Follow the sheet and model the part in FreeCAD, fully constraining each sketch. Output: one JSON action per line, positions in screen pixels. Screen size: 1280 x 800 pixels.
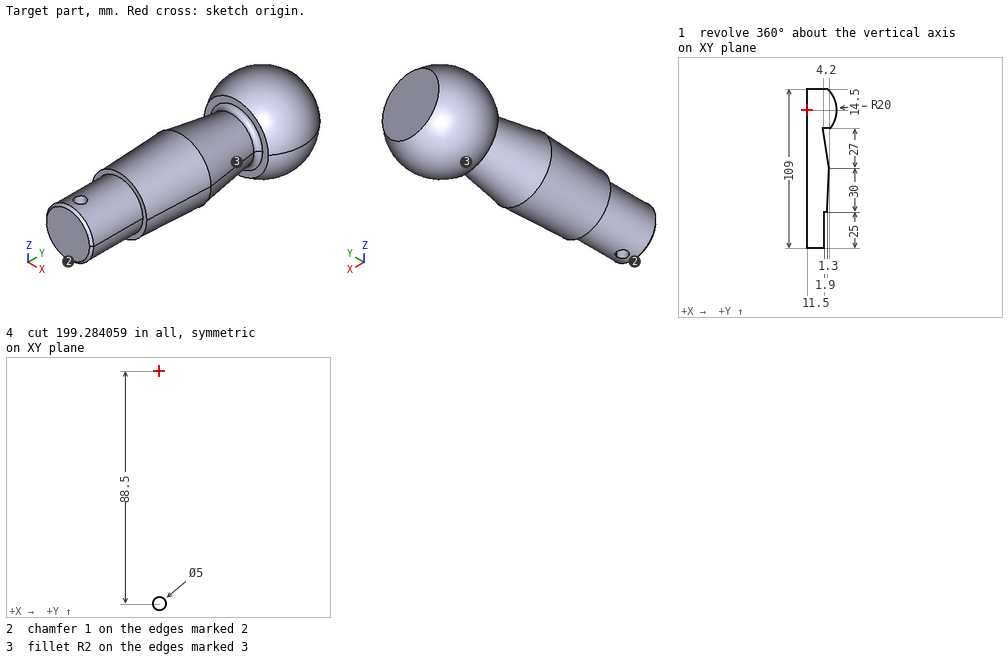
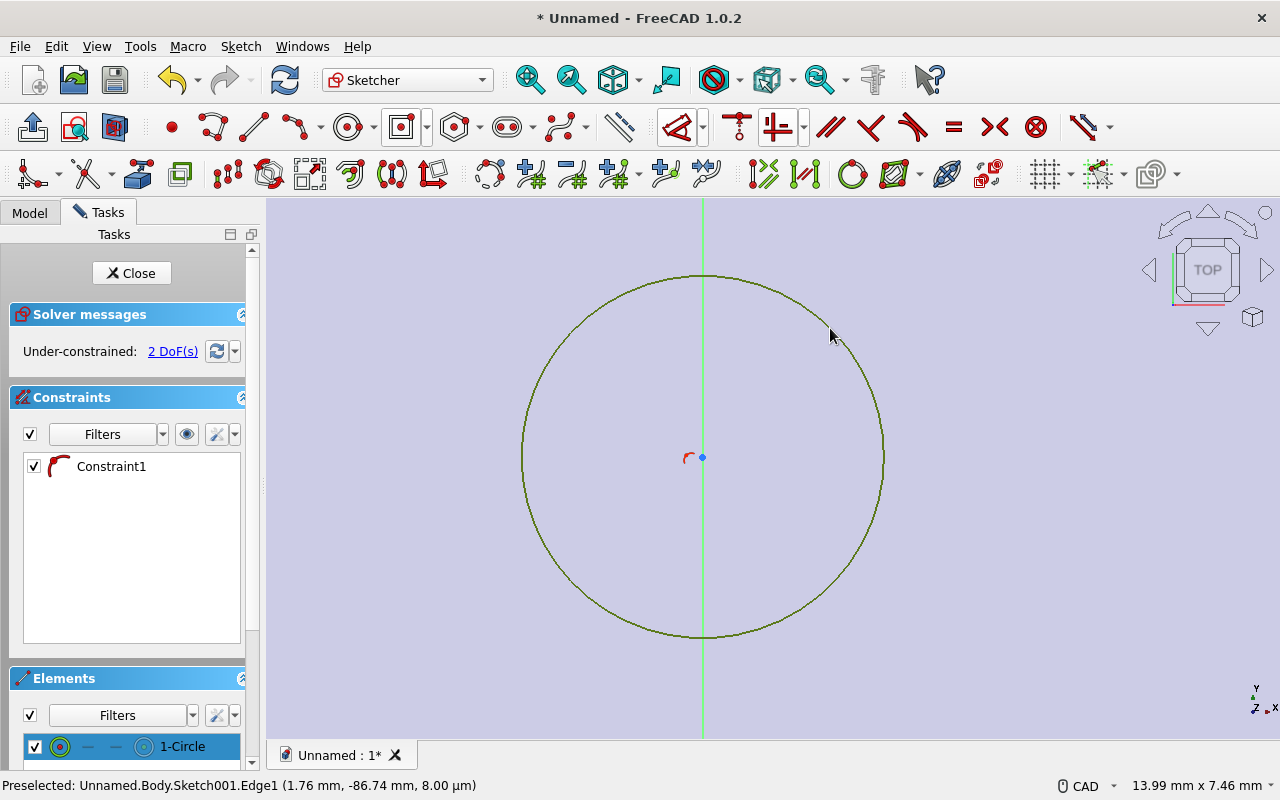
{"action": "left_click", "coordinate": [702, 128]}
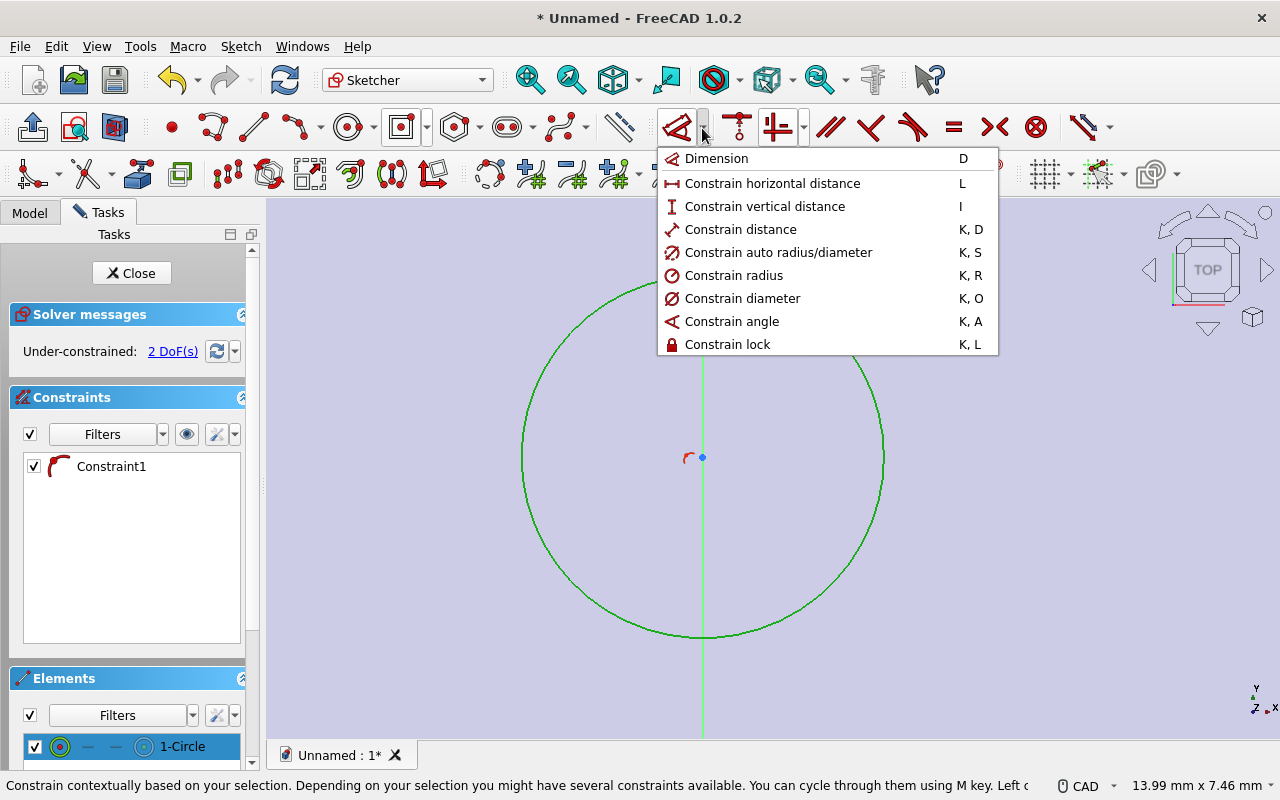
{"action": "left_click", "coordinate": [828, 298]}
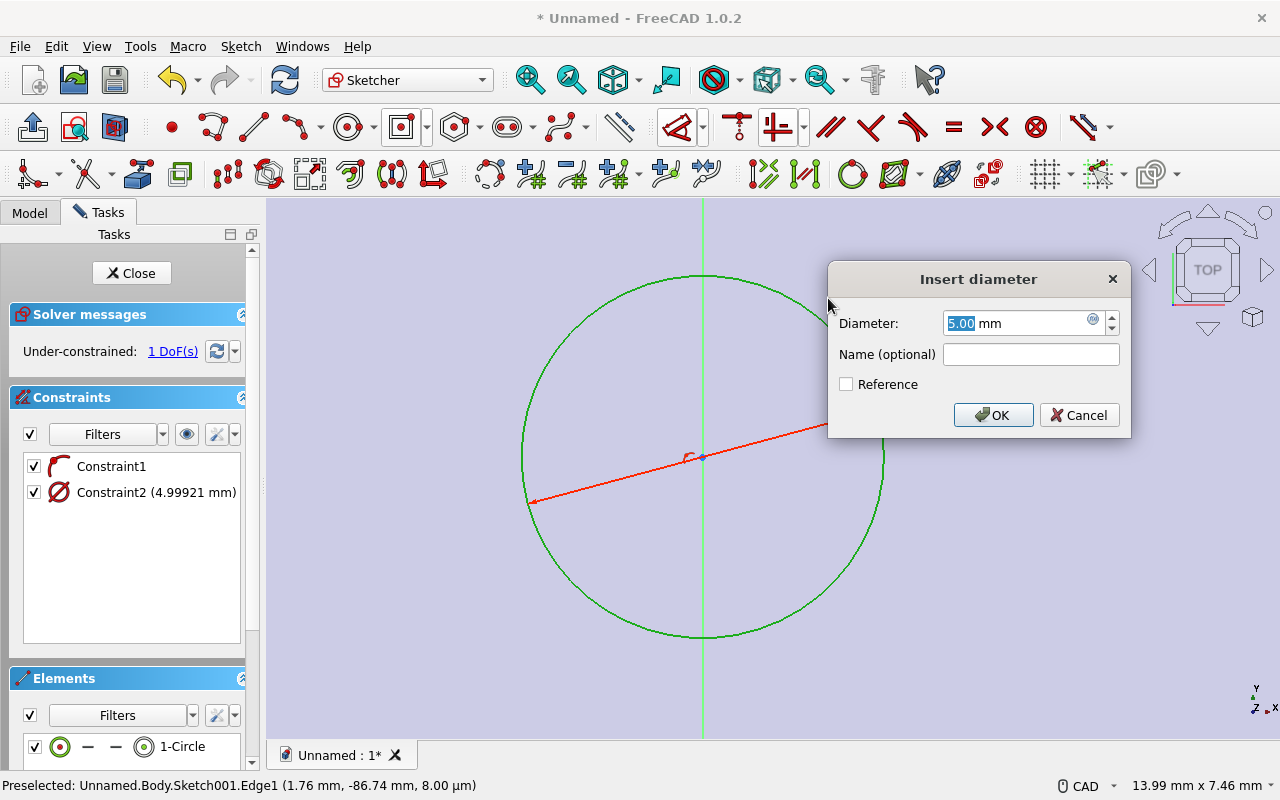
{"action": "type", "text": "5"}
{"action": "key", "text": "Return"}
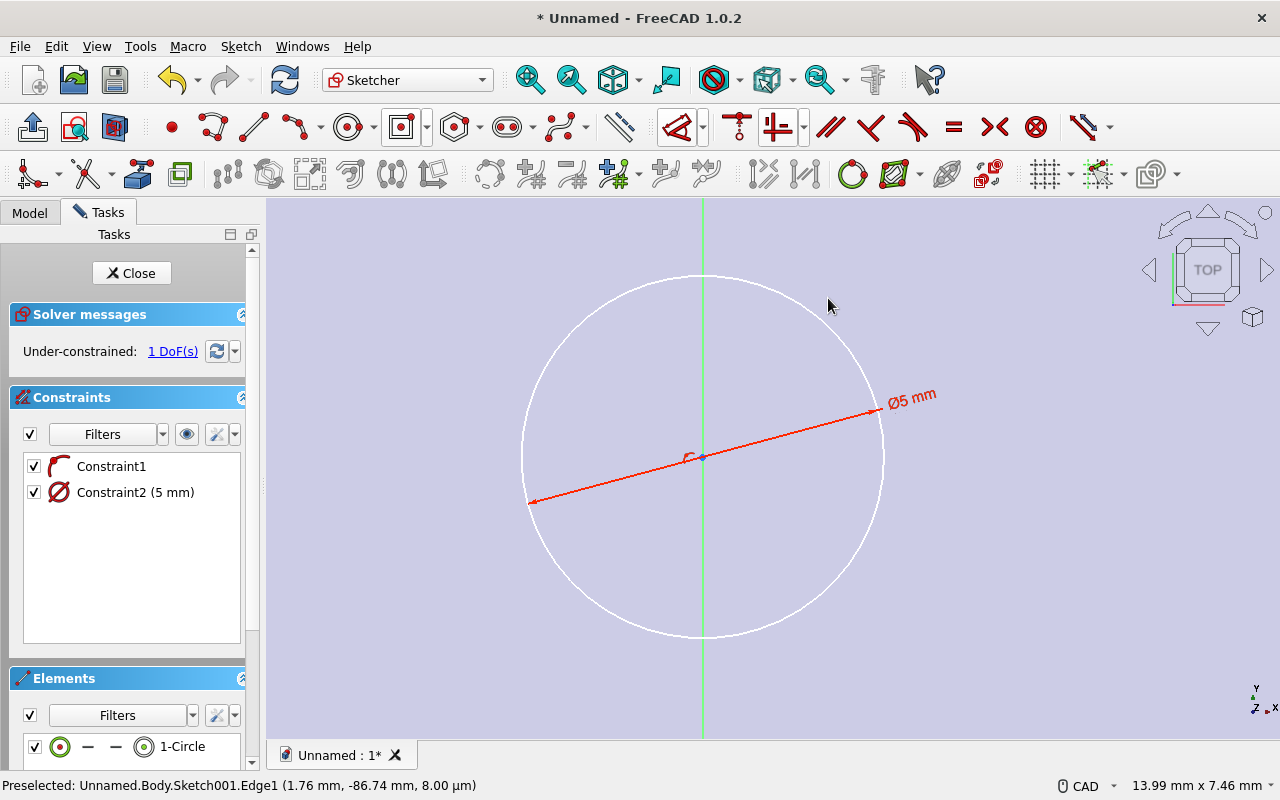
{"action": "left_click", "coordinate": [703, 457]}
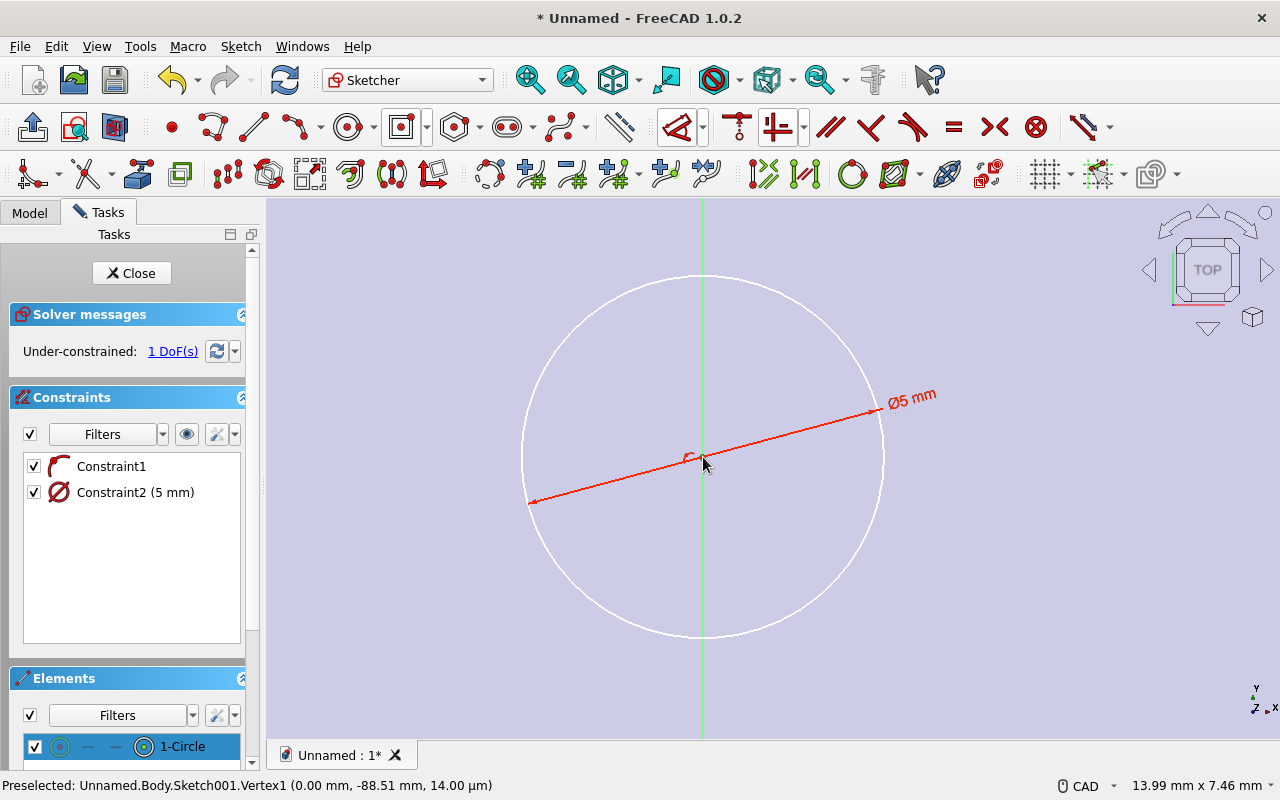
{"action": "left_click", "coordinate": [702, 128]}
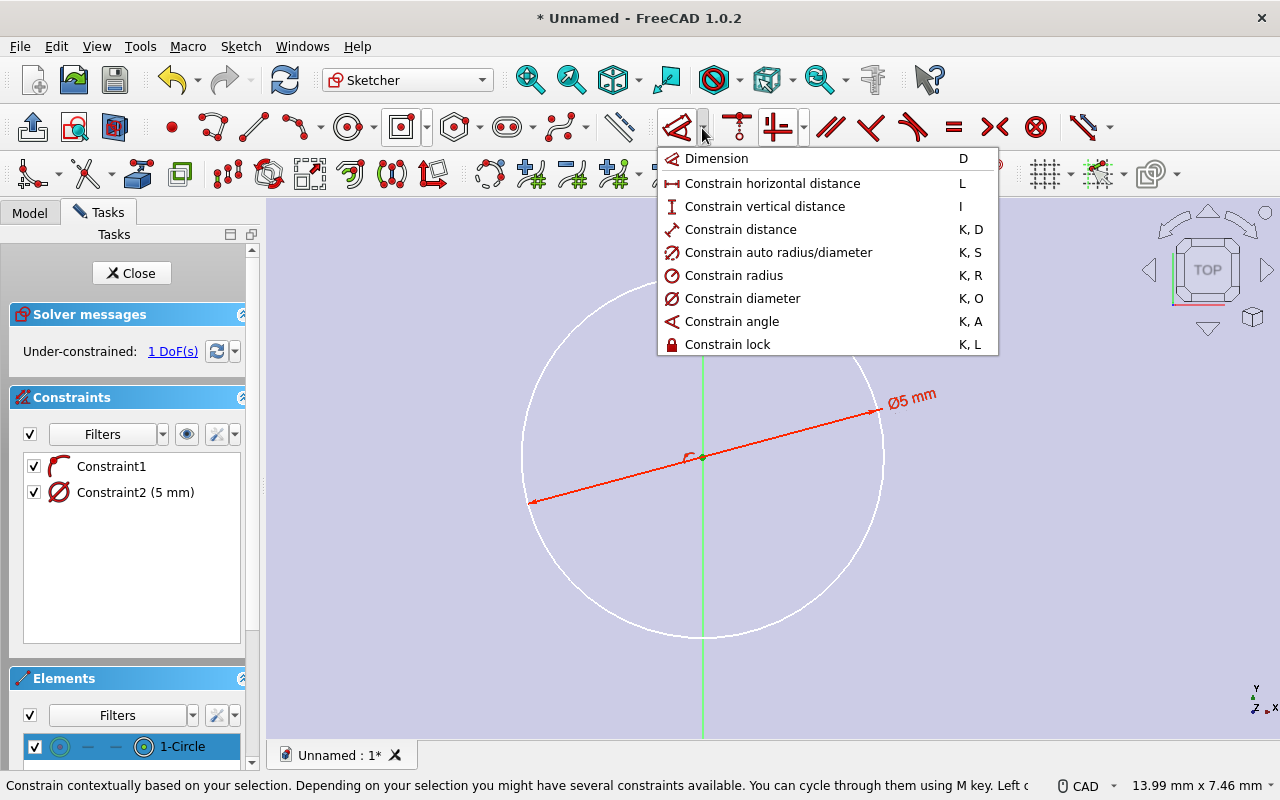
{"action": "left_click", "coordinate": [828, 206]}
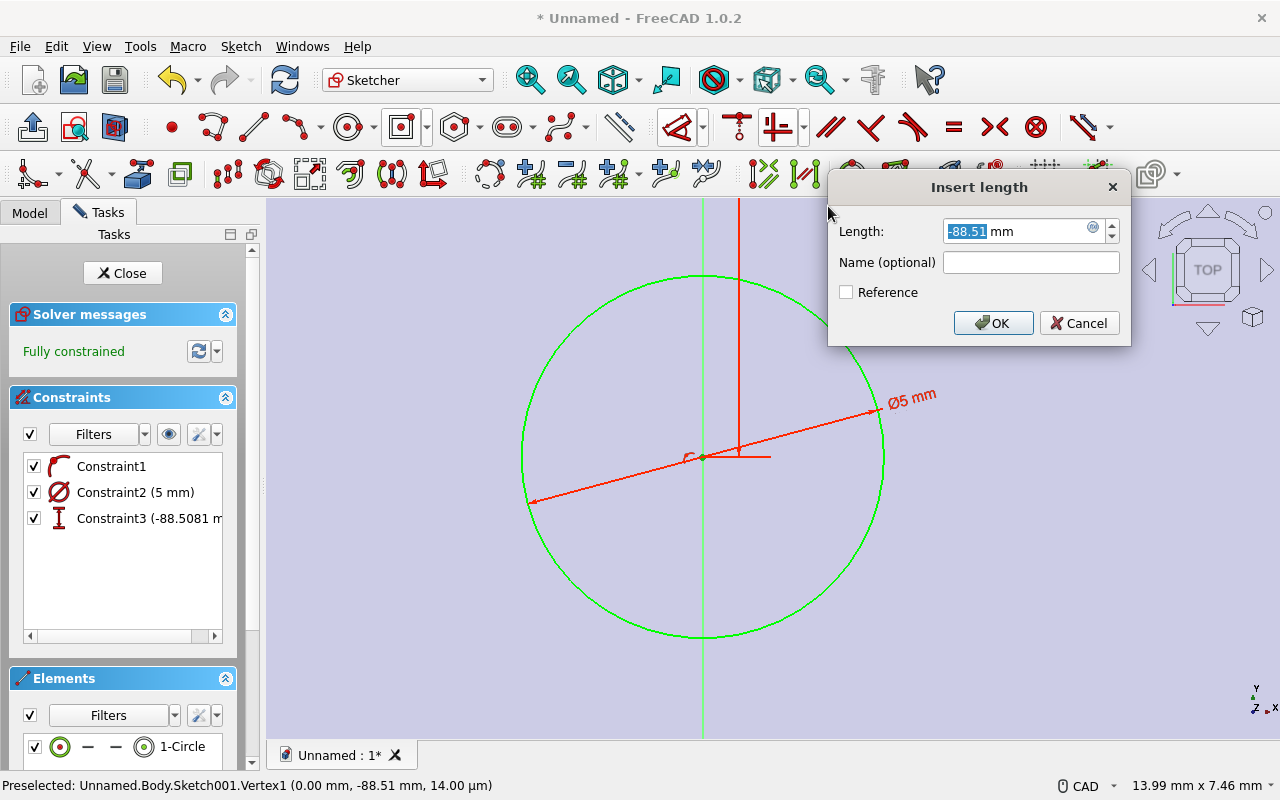
{"action": "type", "text": "-88.5"}
{"action": "key", "text": "Return"}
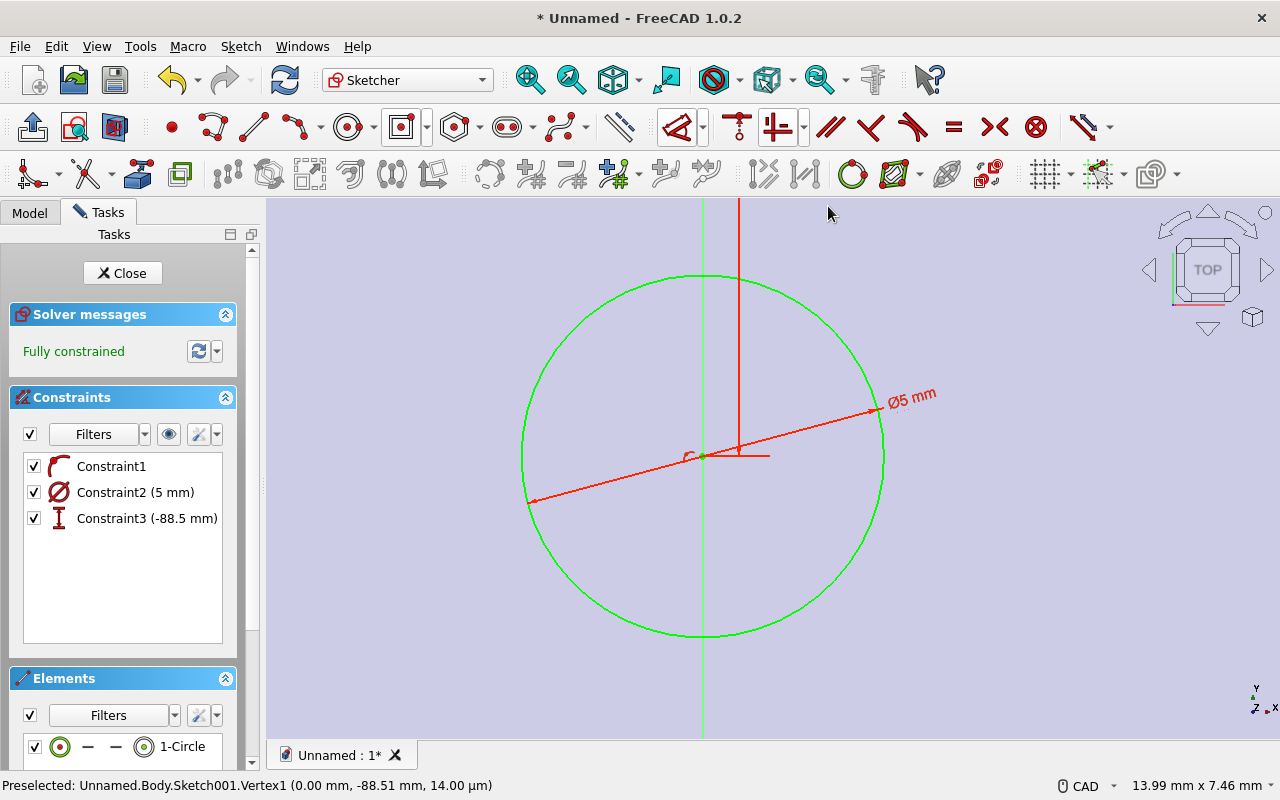
{"action": "left_click", "coordinate": [123, 273]}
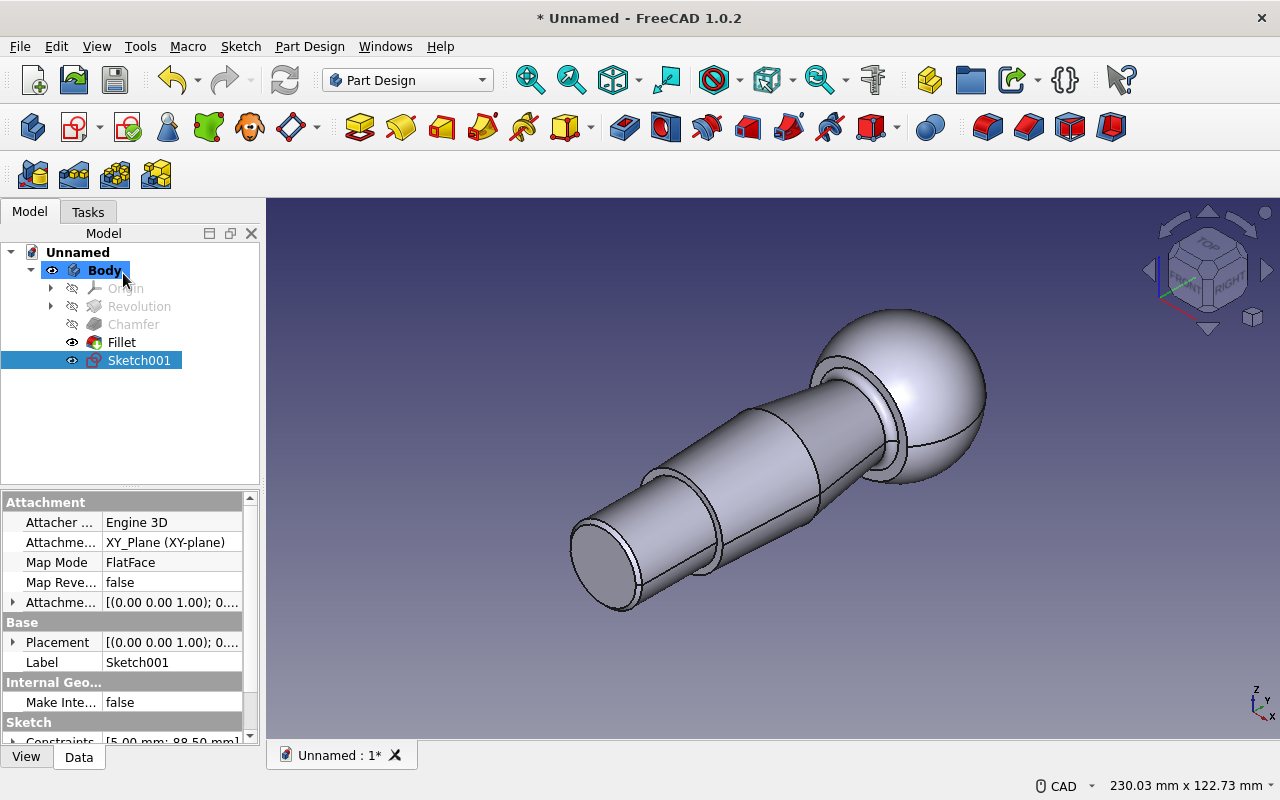
{"action": "left_click", "coordinate": [625, 128]}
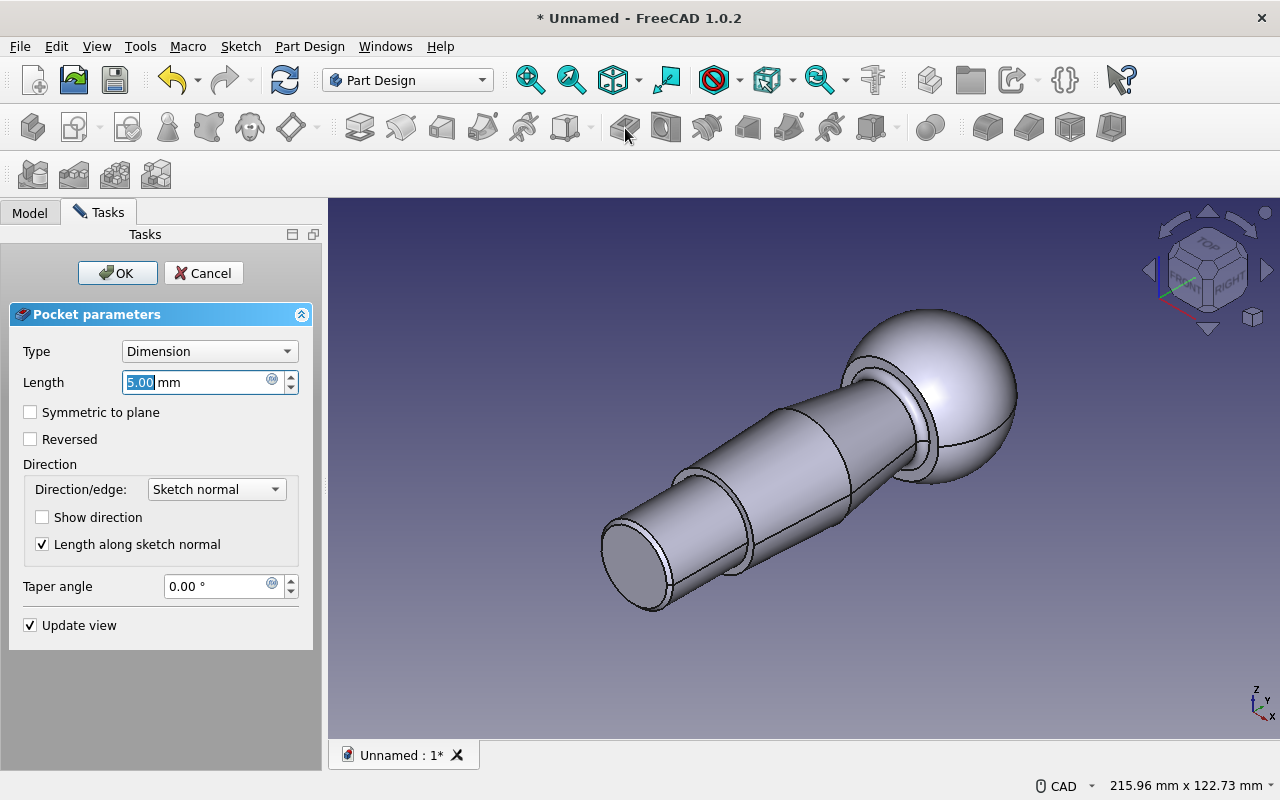
{"action": "type", "text": "199.284059"}
{"action": "key", "text": "Tab"}